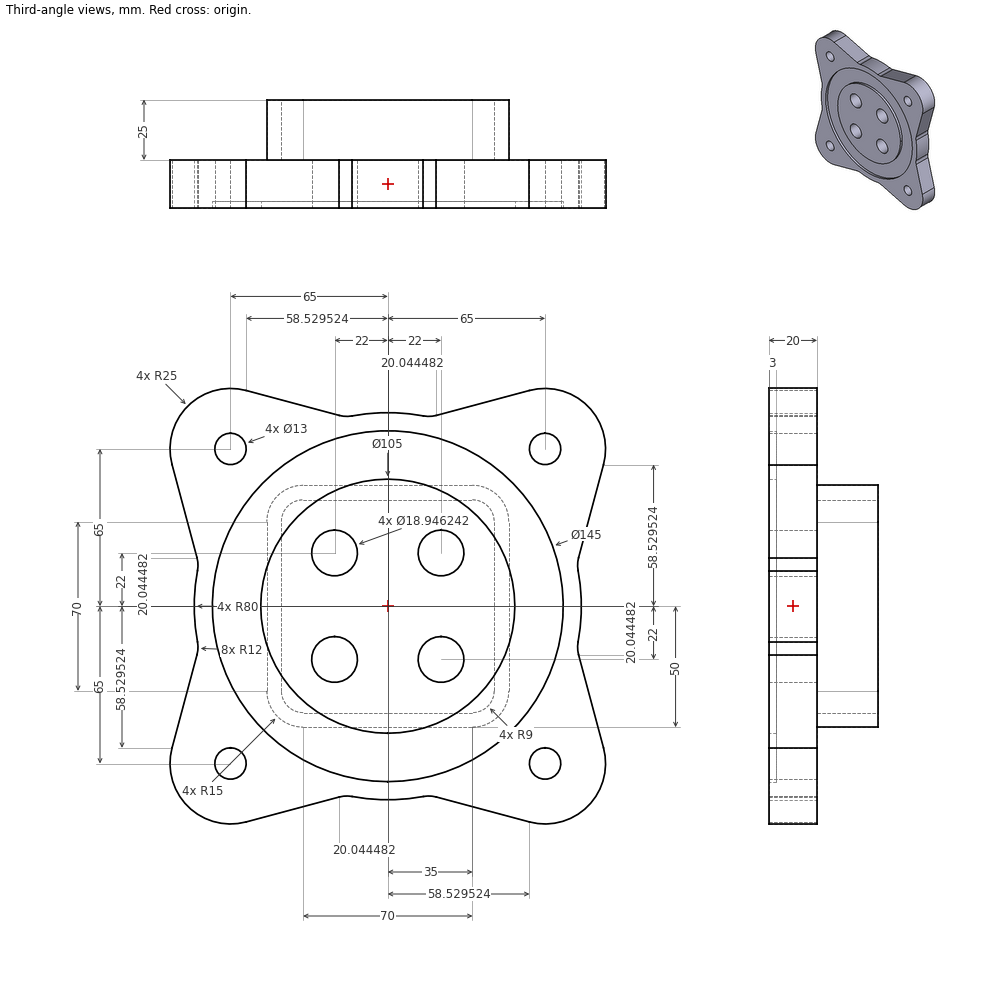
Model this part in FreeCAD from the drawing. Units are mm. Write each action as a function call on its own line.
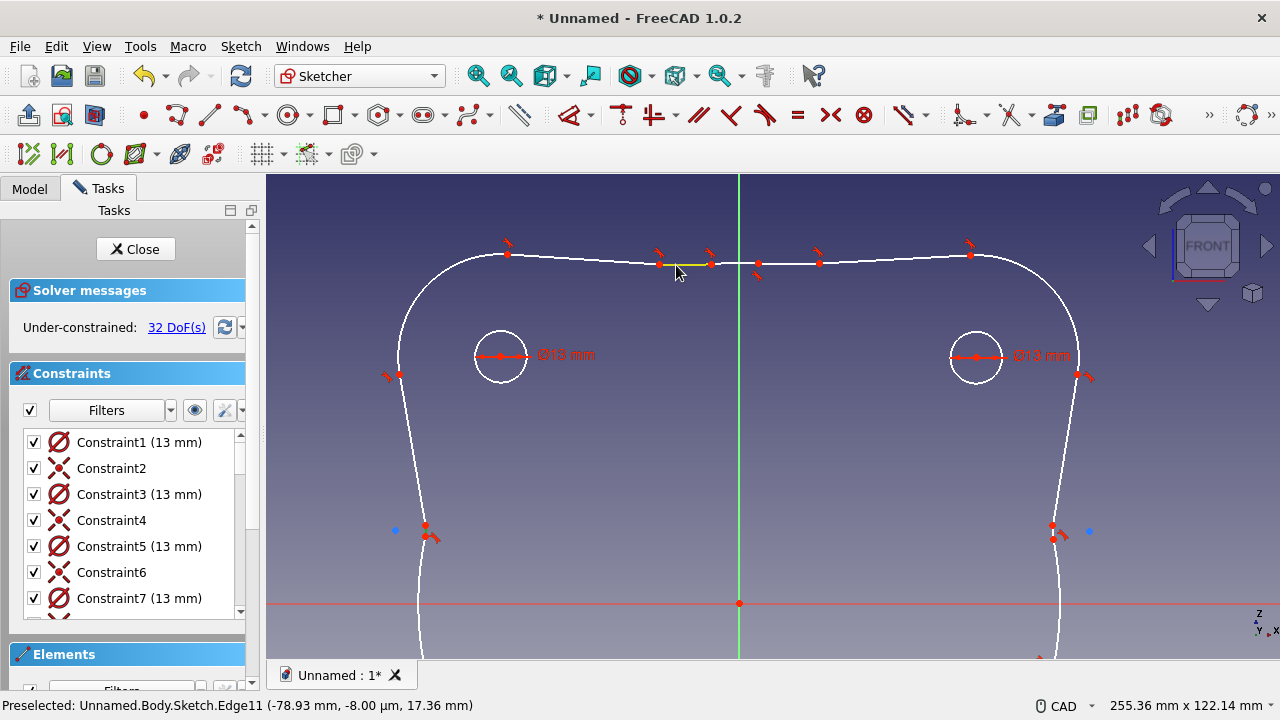
click(675, 265)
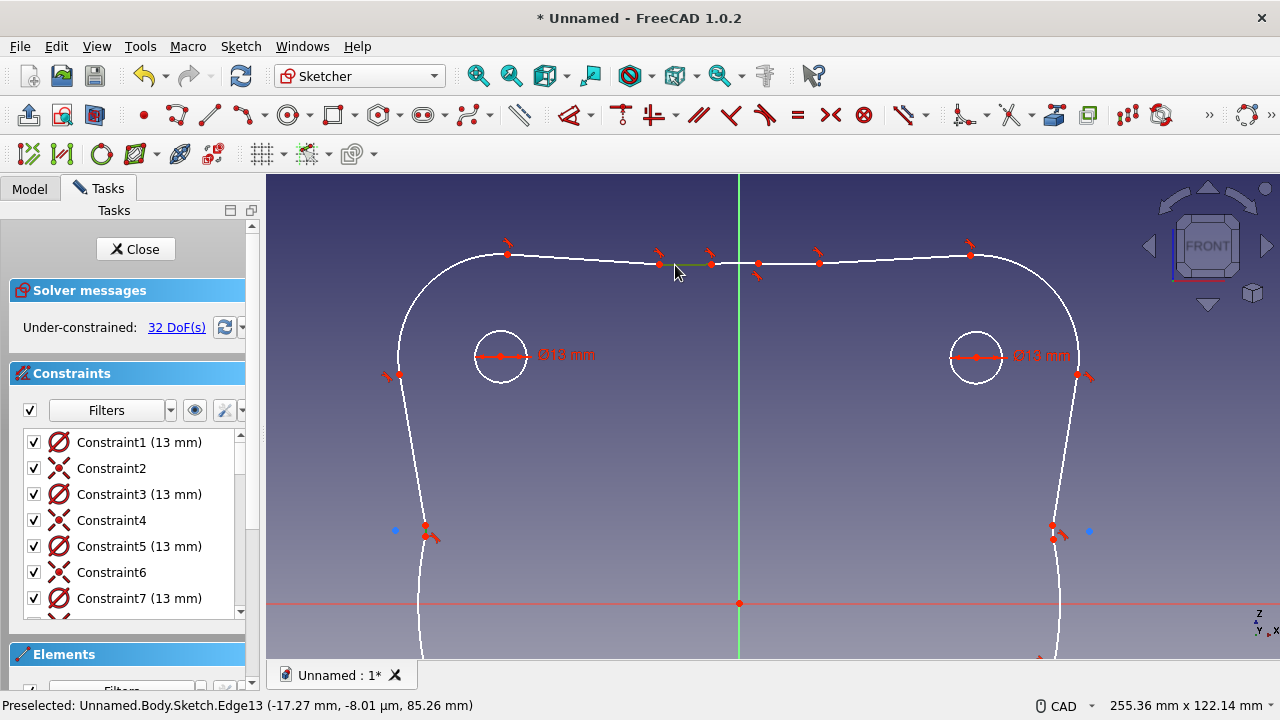
click(777, 264)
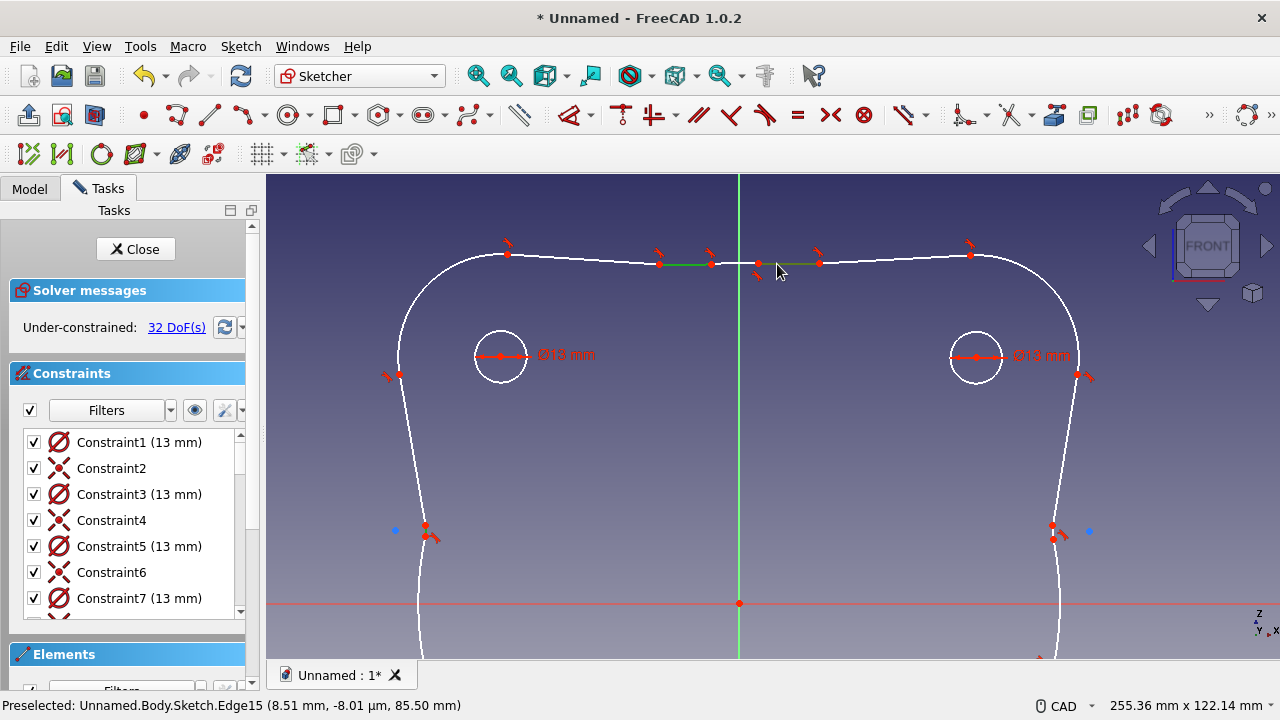
scroll(1053, 532, up, 4)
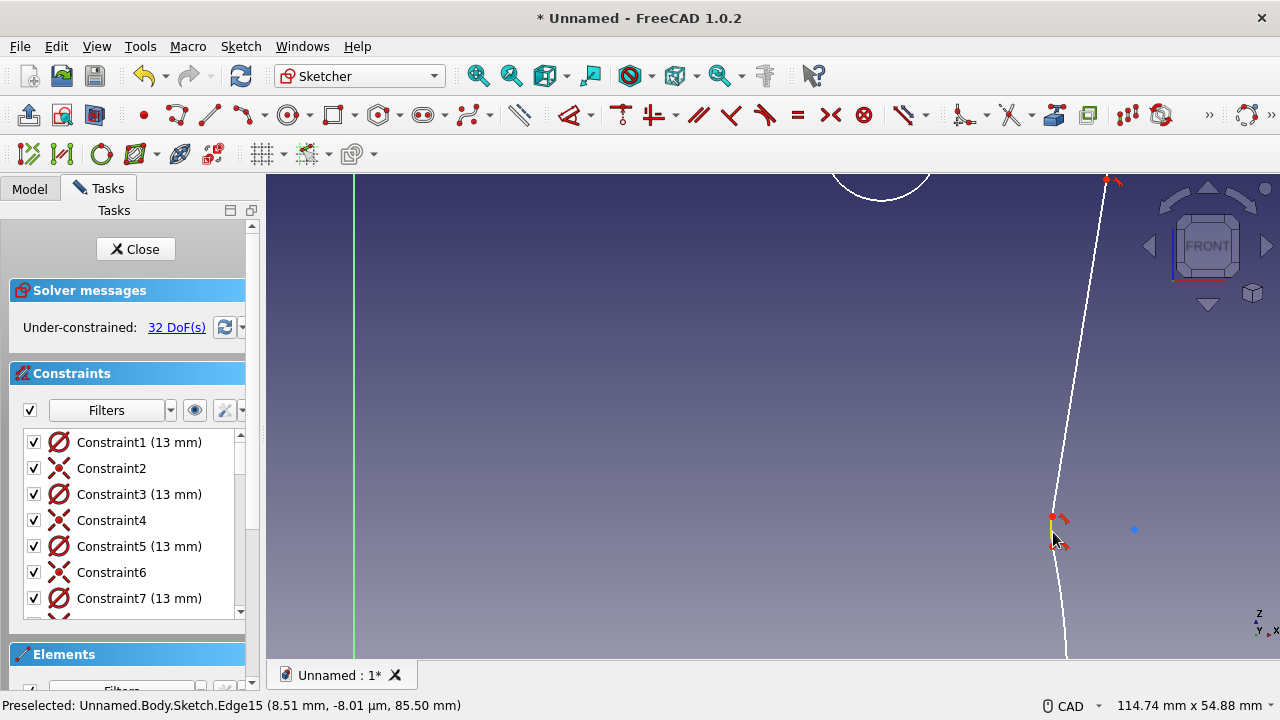
click(1051, 532)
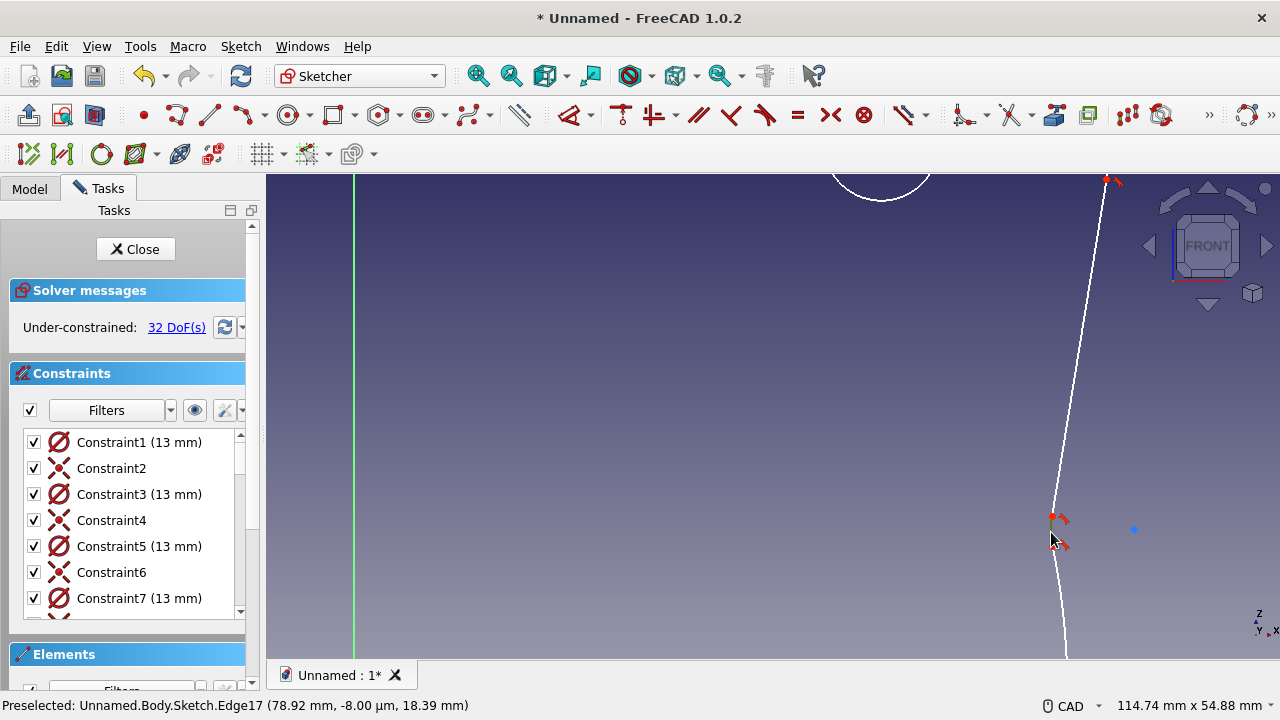
scroll(793, 347, down, 8)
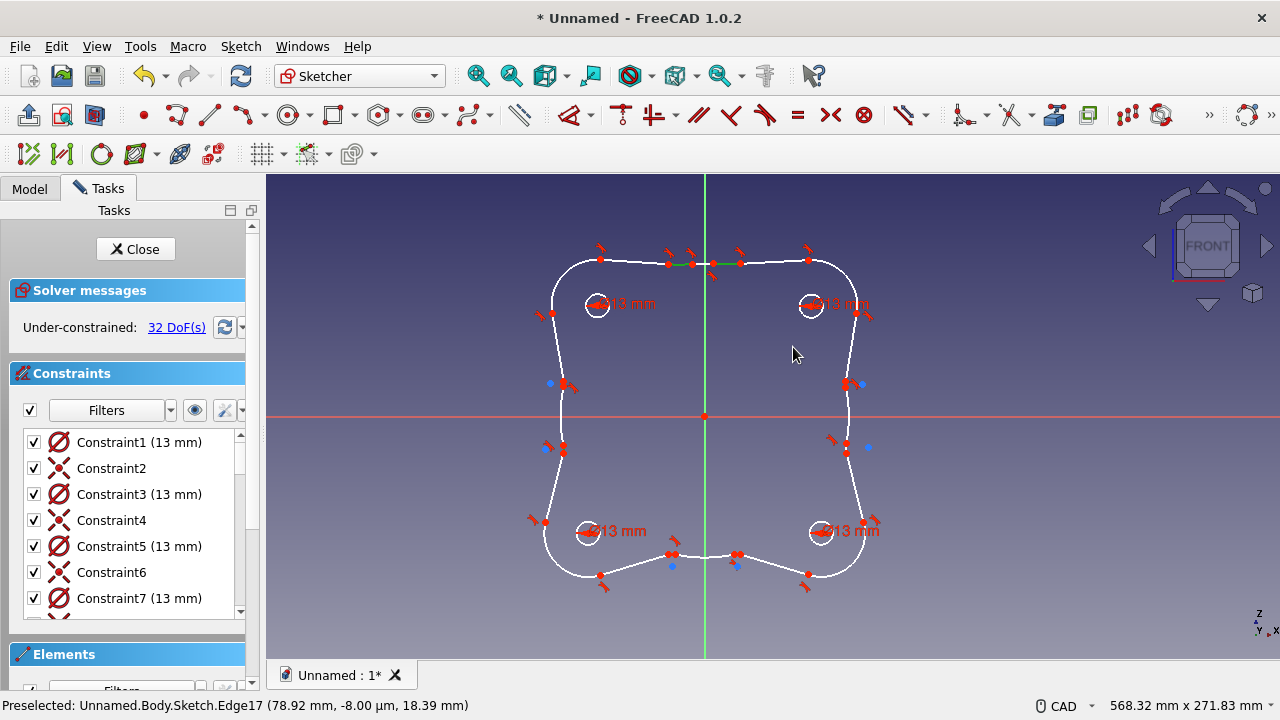
scroll(846, 447, up, 8)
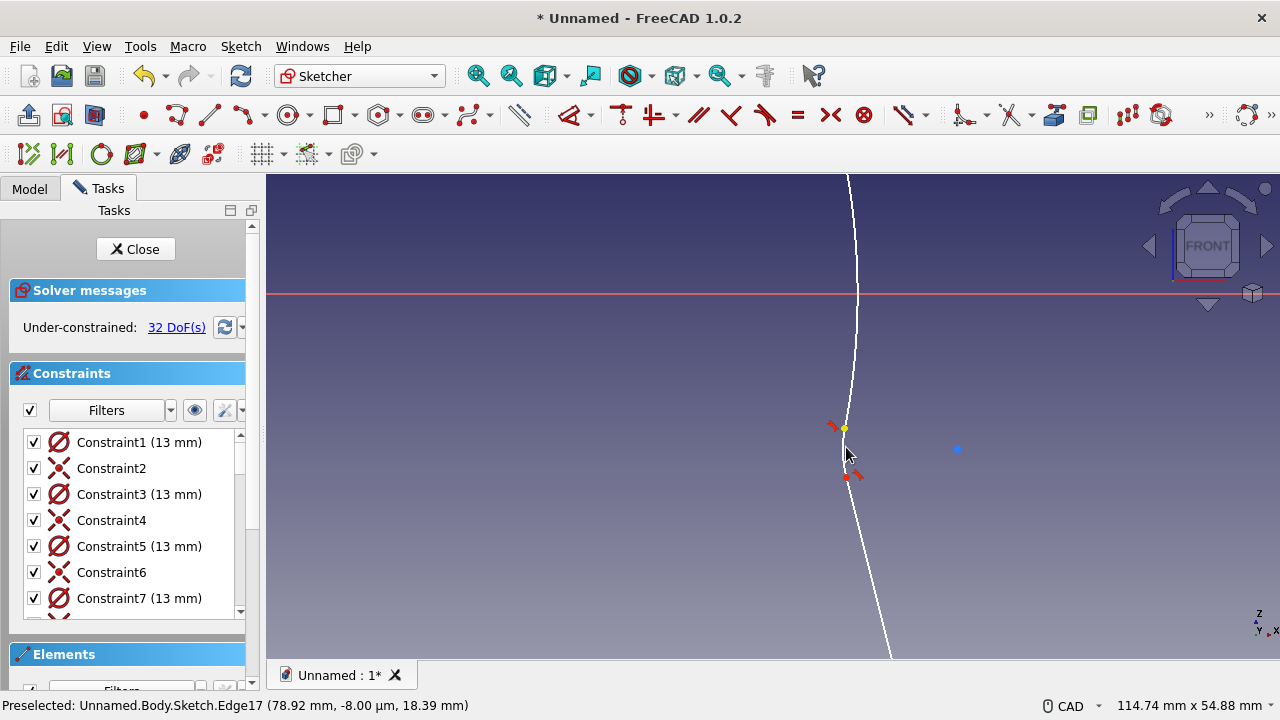
click(843, 443)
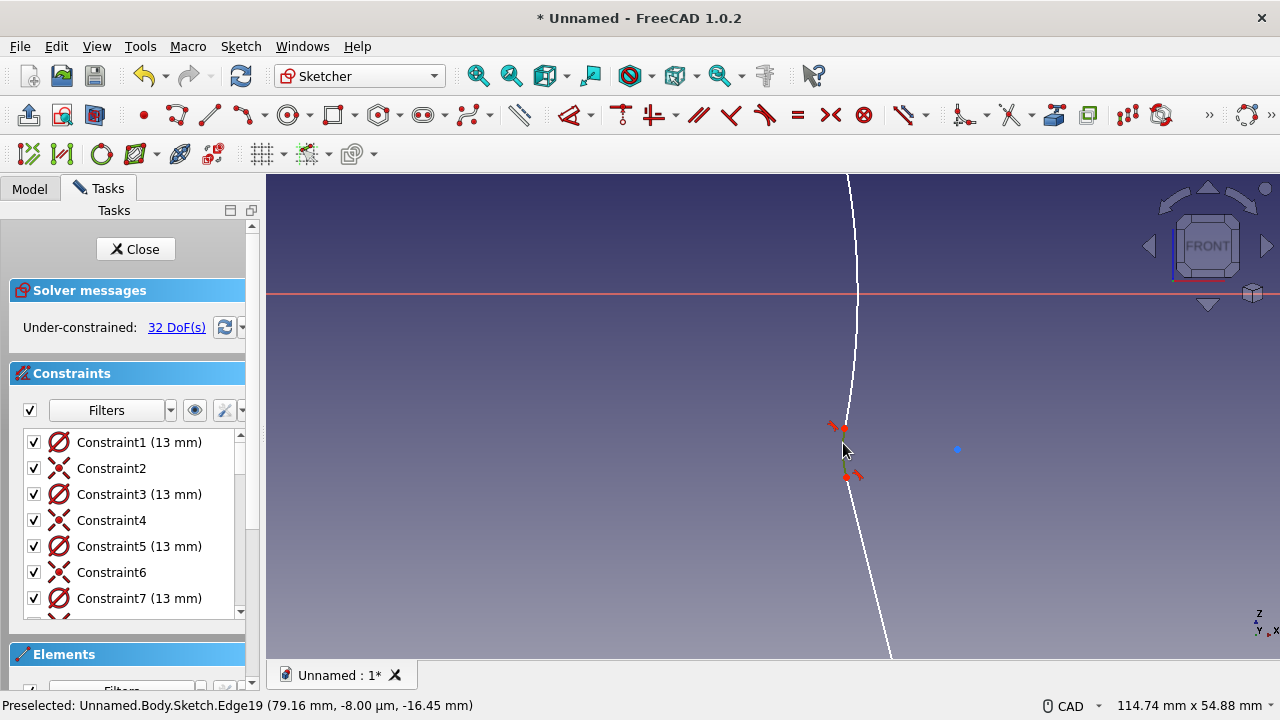
scroll(846, 447, down, 8)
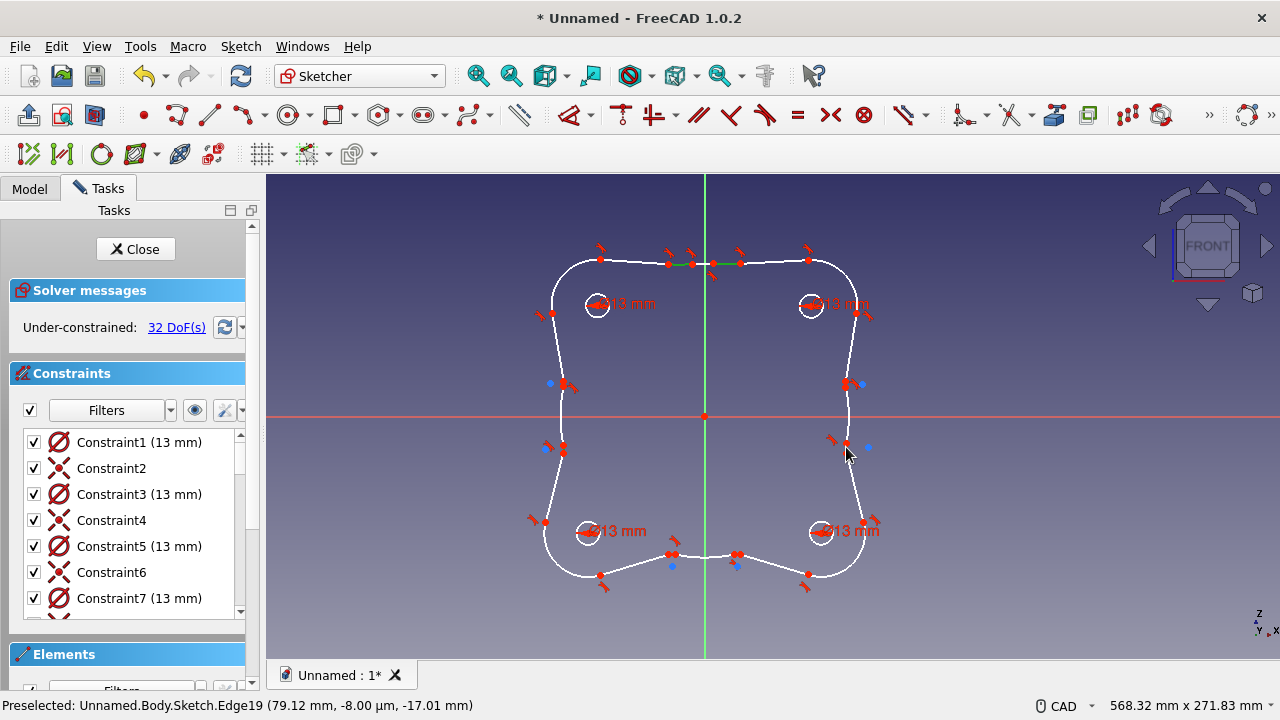
scroll(739, 554, up, 11)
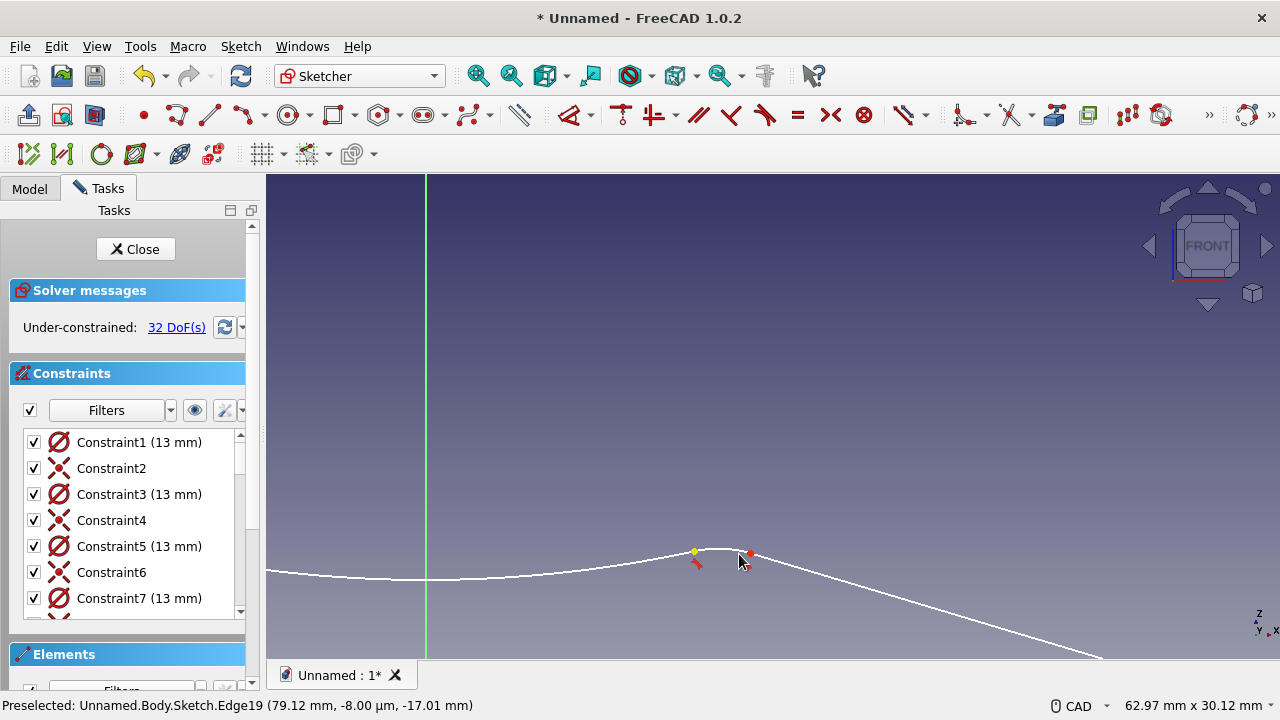
click(734, 550)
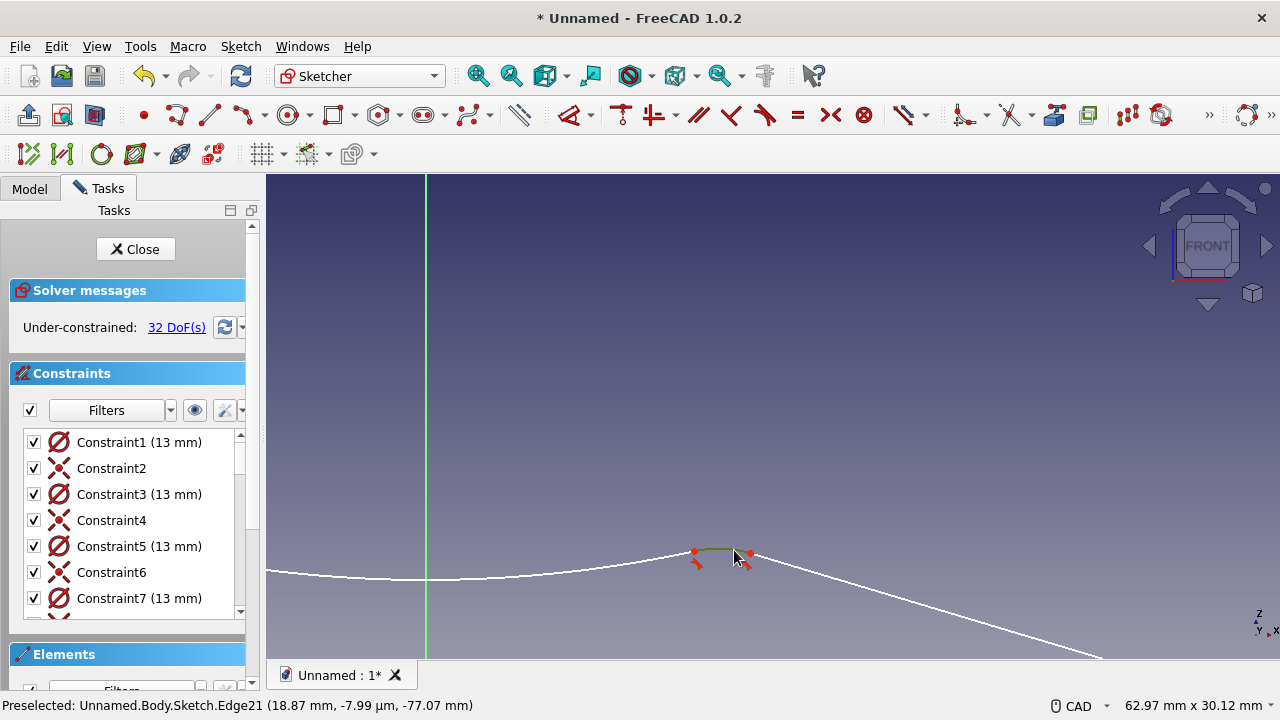
scroll(739, 555, down, 11)